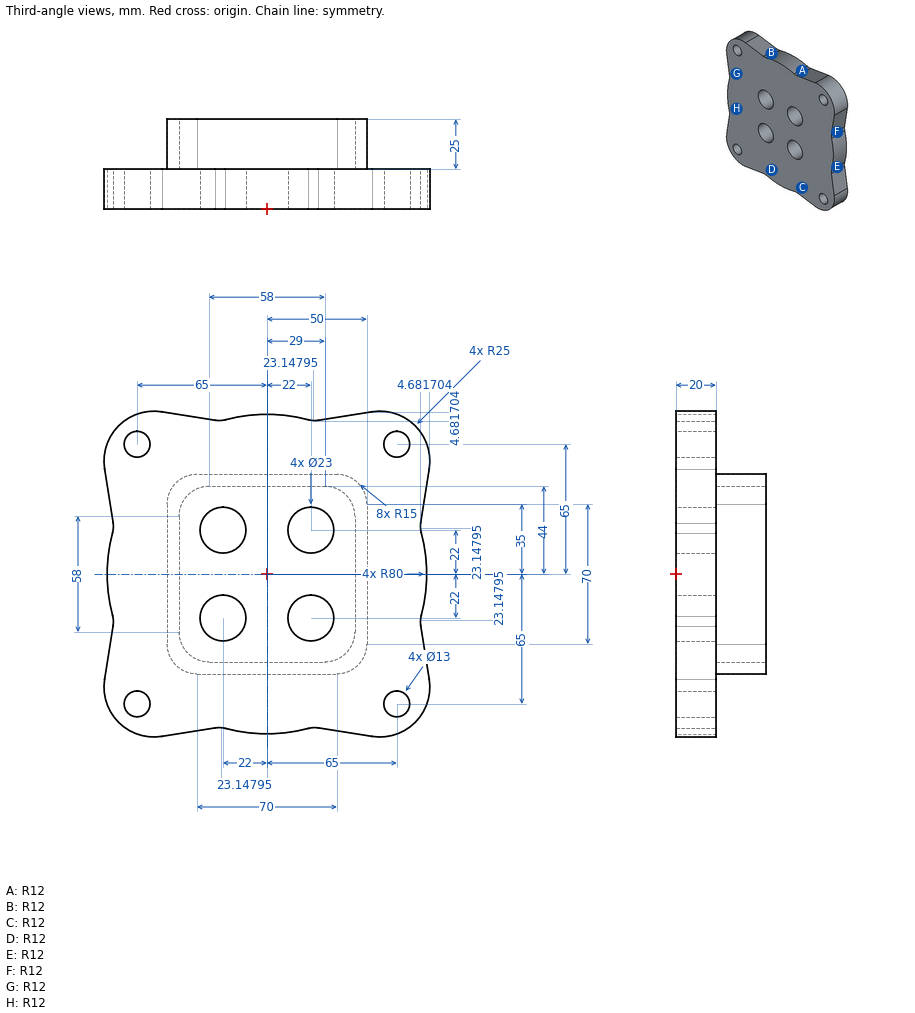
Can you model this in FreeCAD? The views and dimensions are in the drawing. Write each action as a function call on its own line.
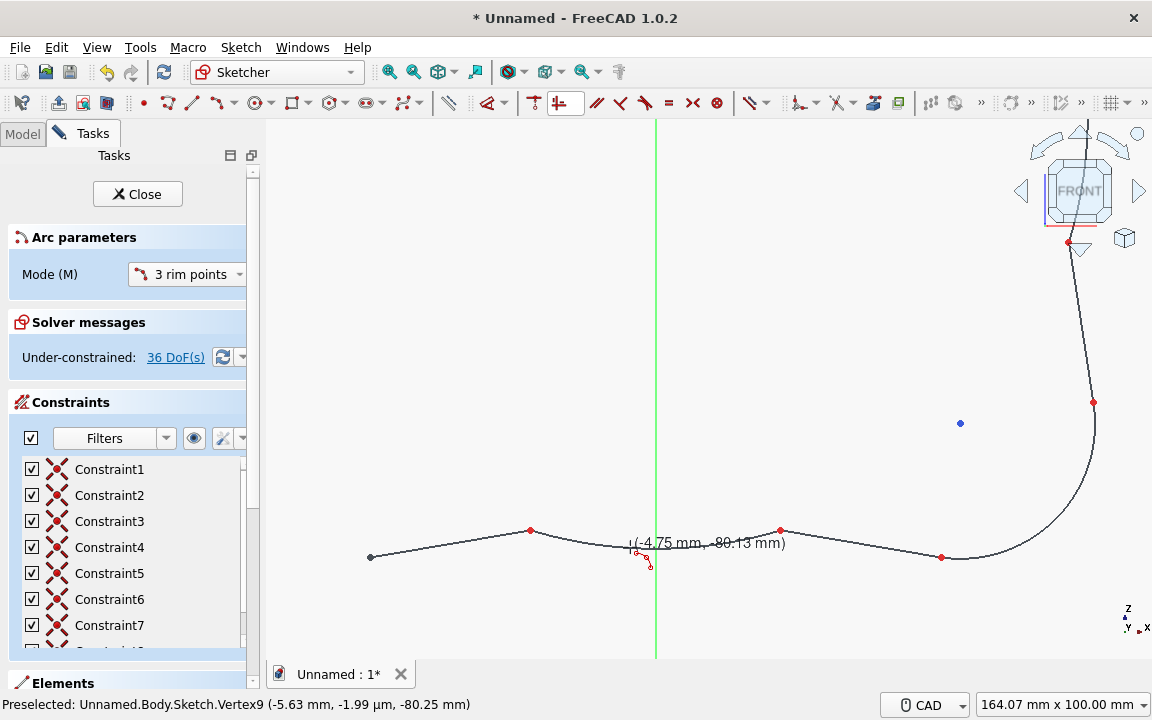
click(370, 558)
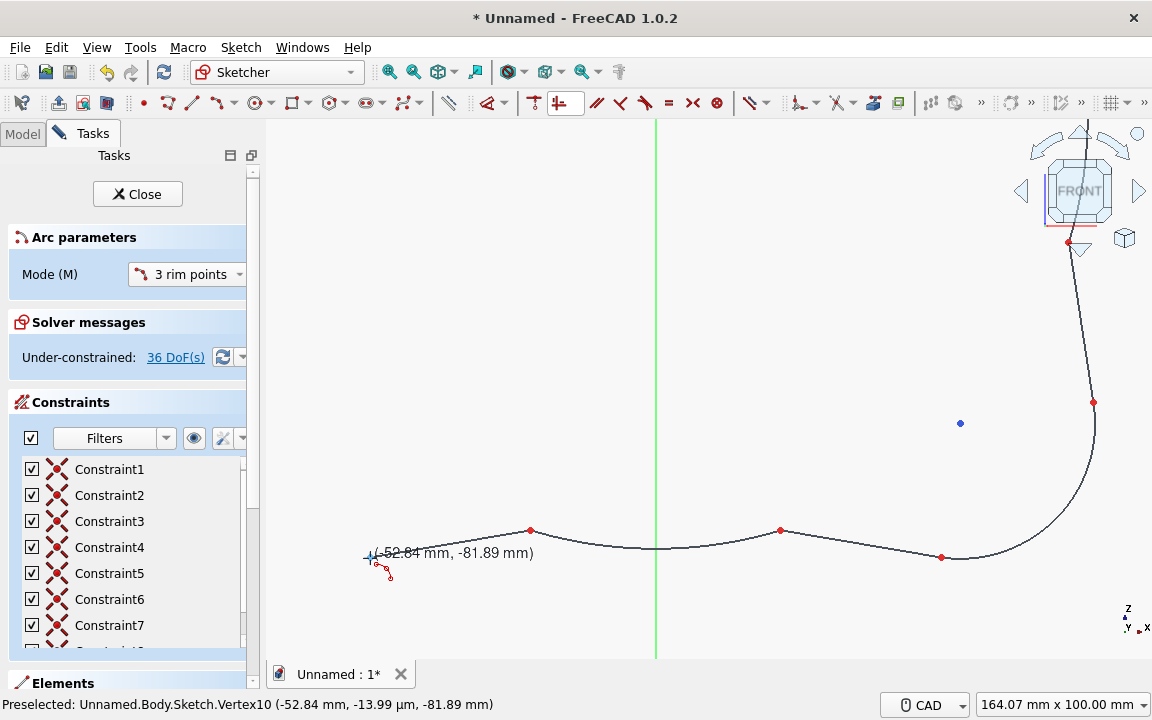
scroll(632, 548, down, 5)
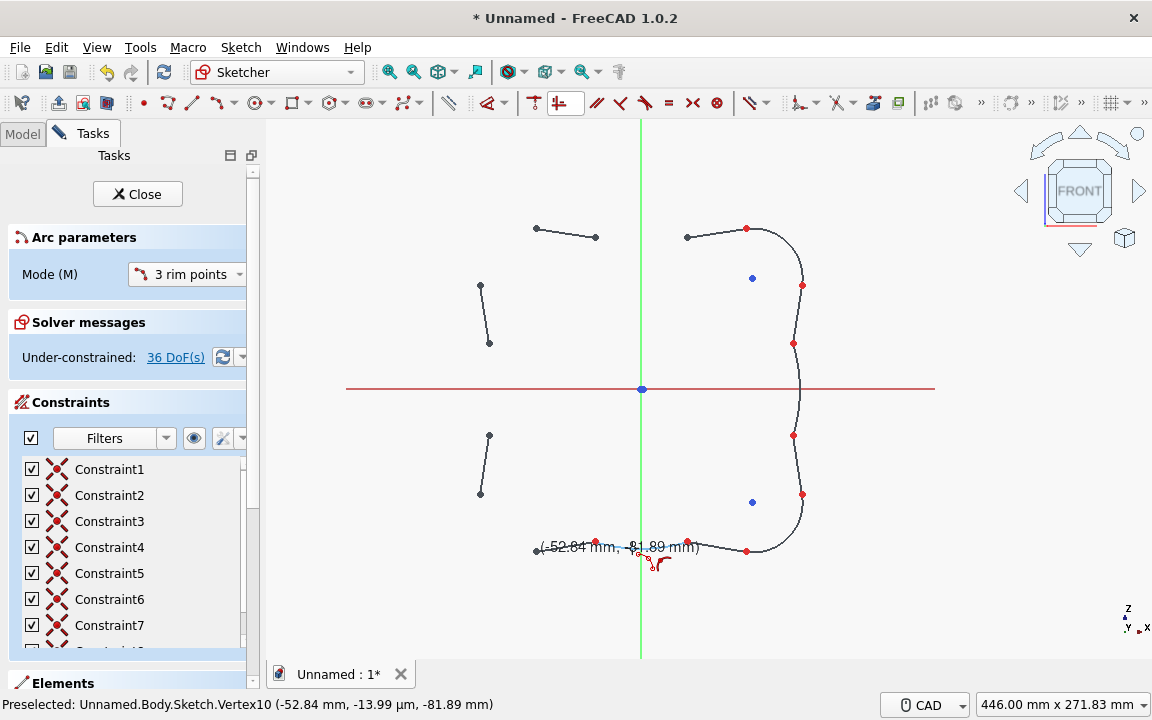
click(480, 495)
click(493, 537)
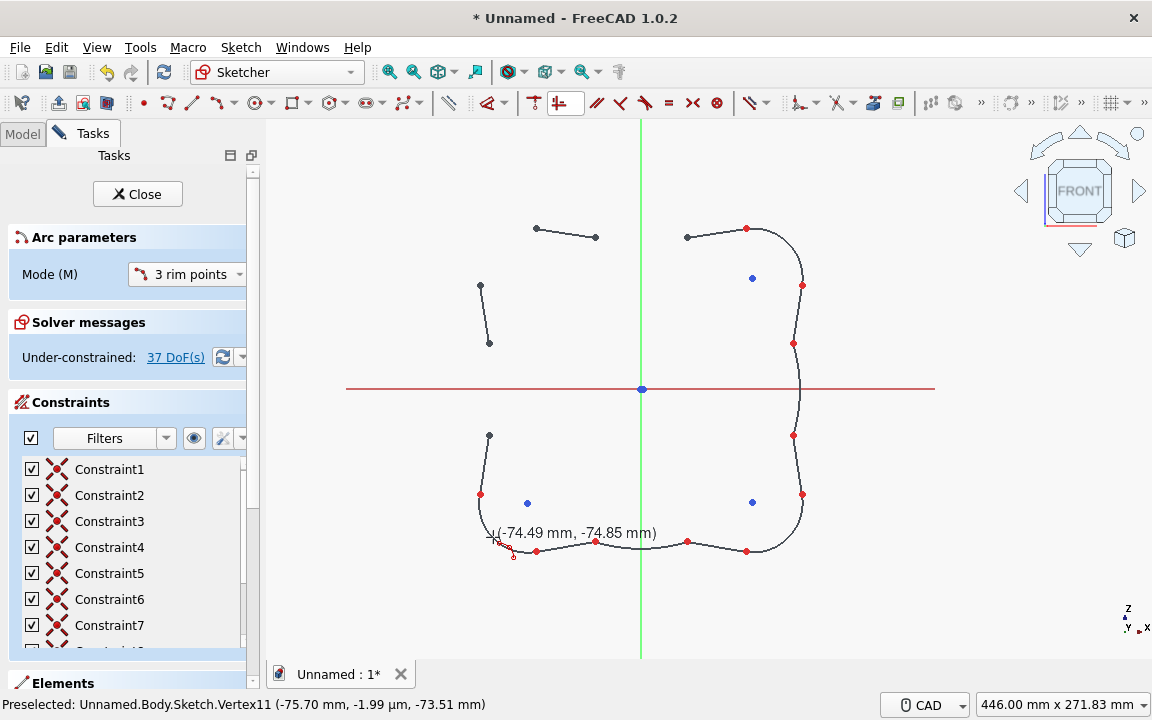
click(489, 436)
click(489, 344)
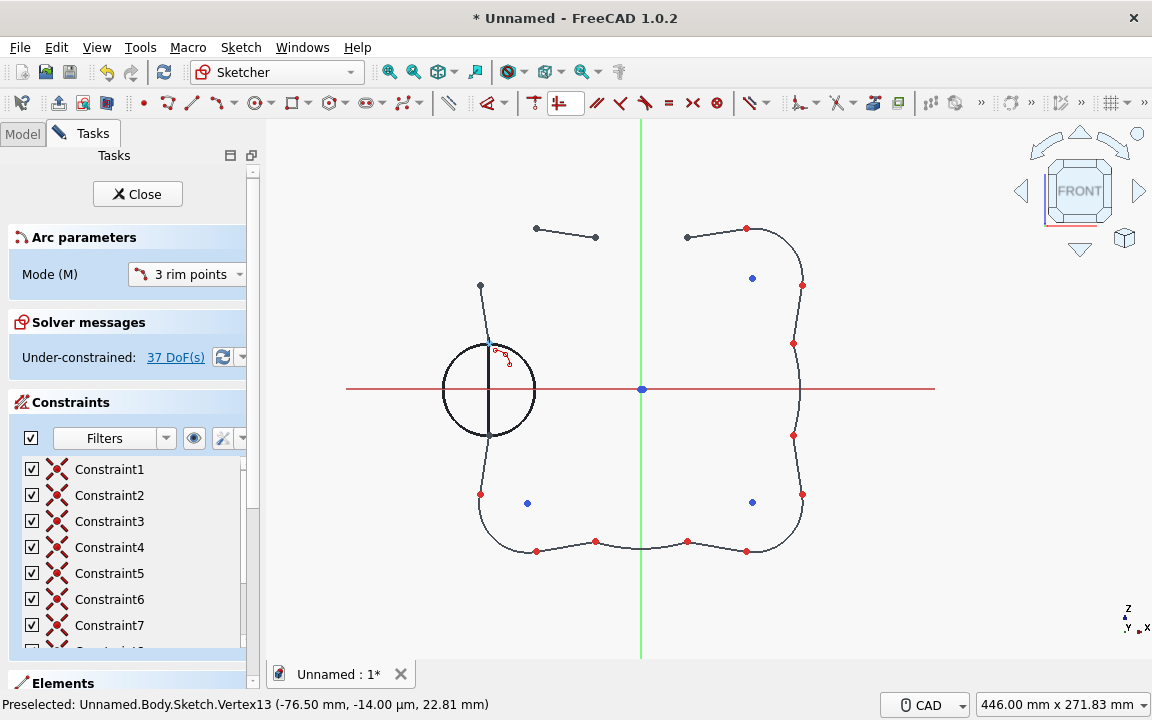
scroll(482, 380, up, 5)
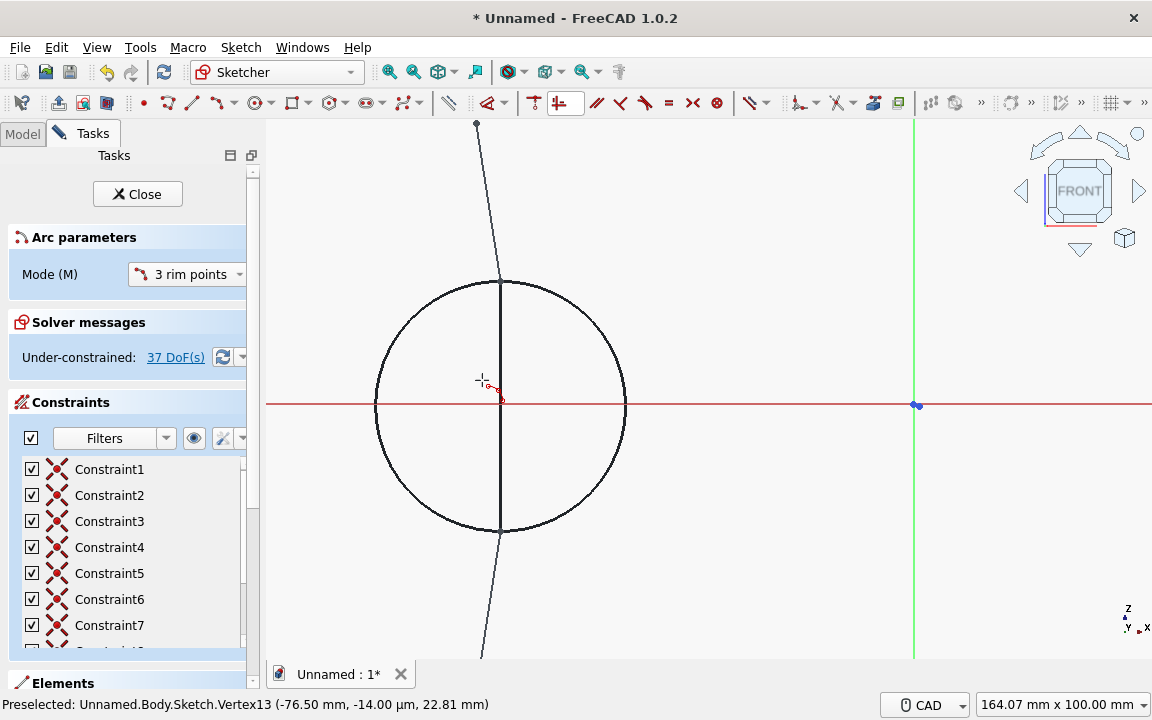
click(482, 379)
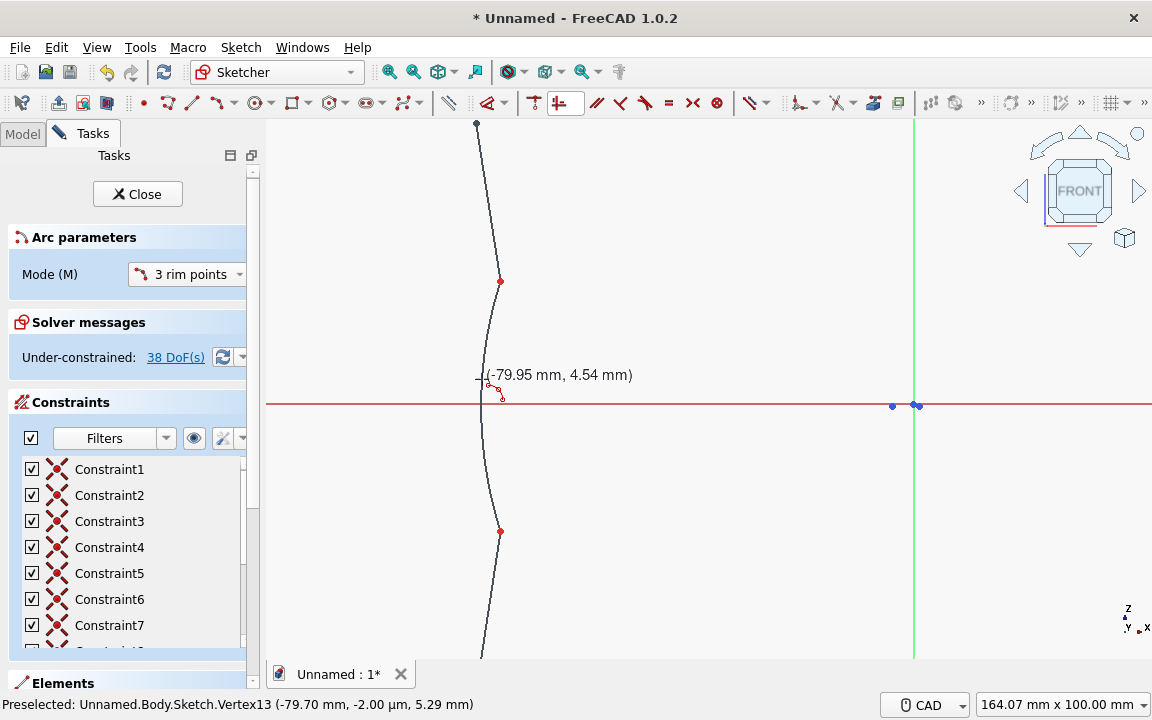
scroll(482, 380, down, 5)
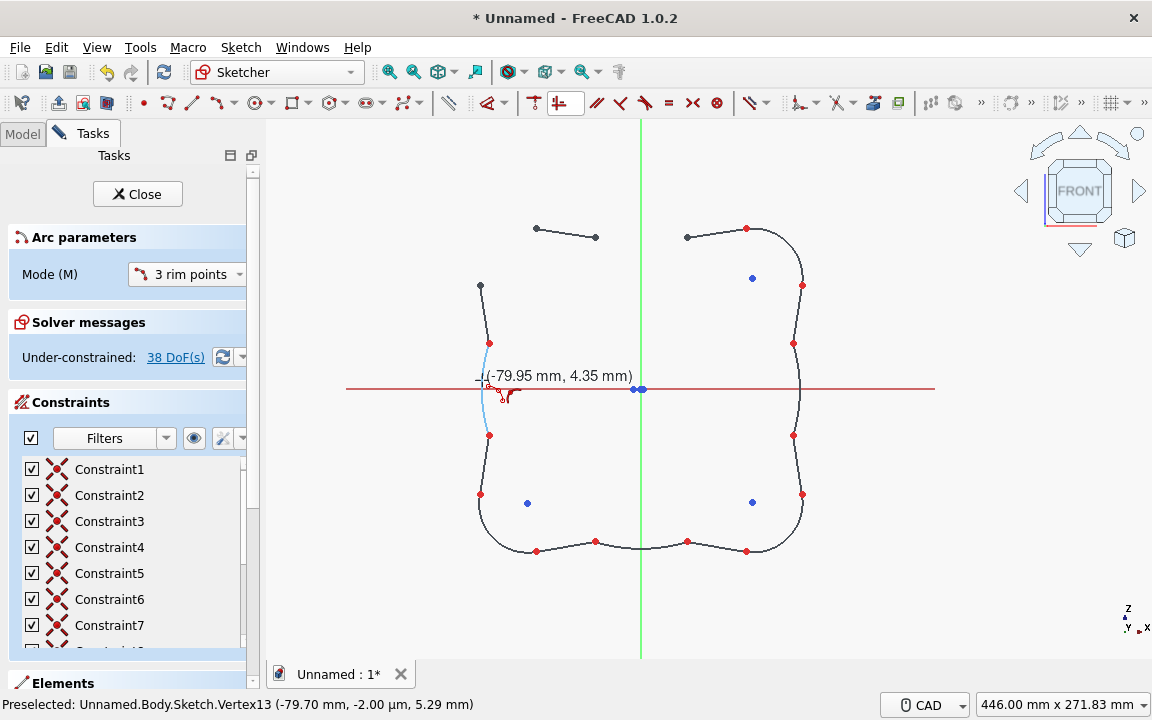
click(480, 286)
click(536, 229)
click(493, 242)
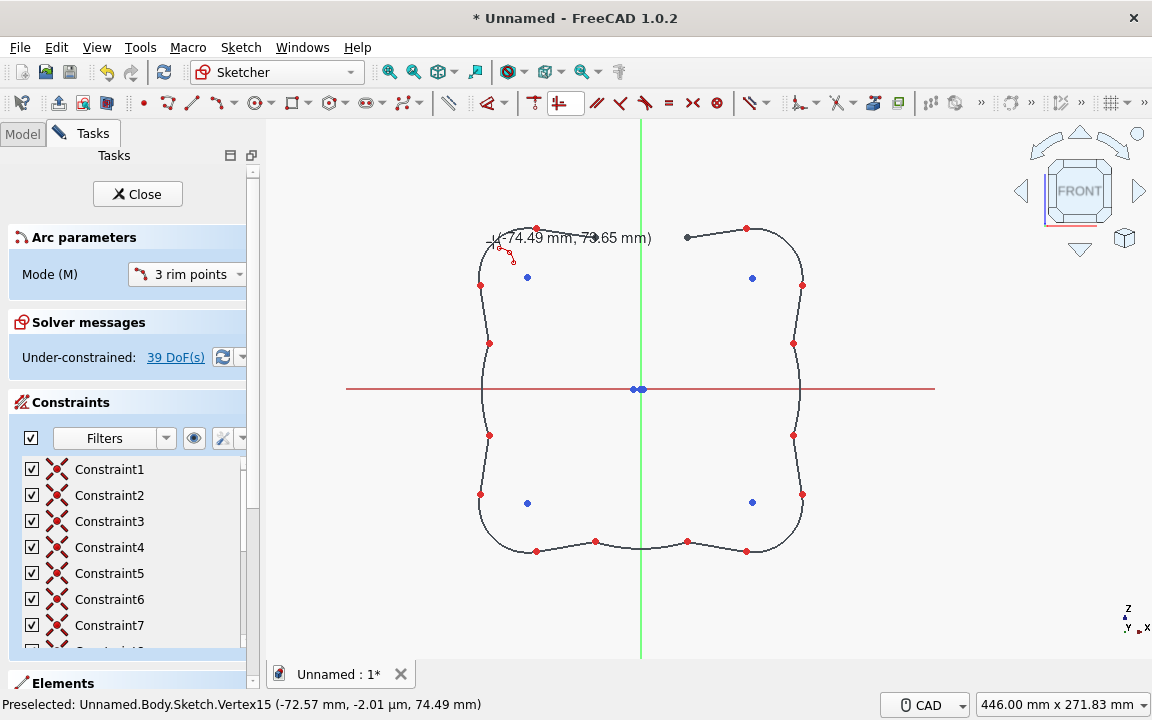
click(595, 238)
click(687, 238)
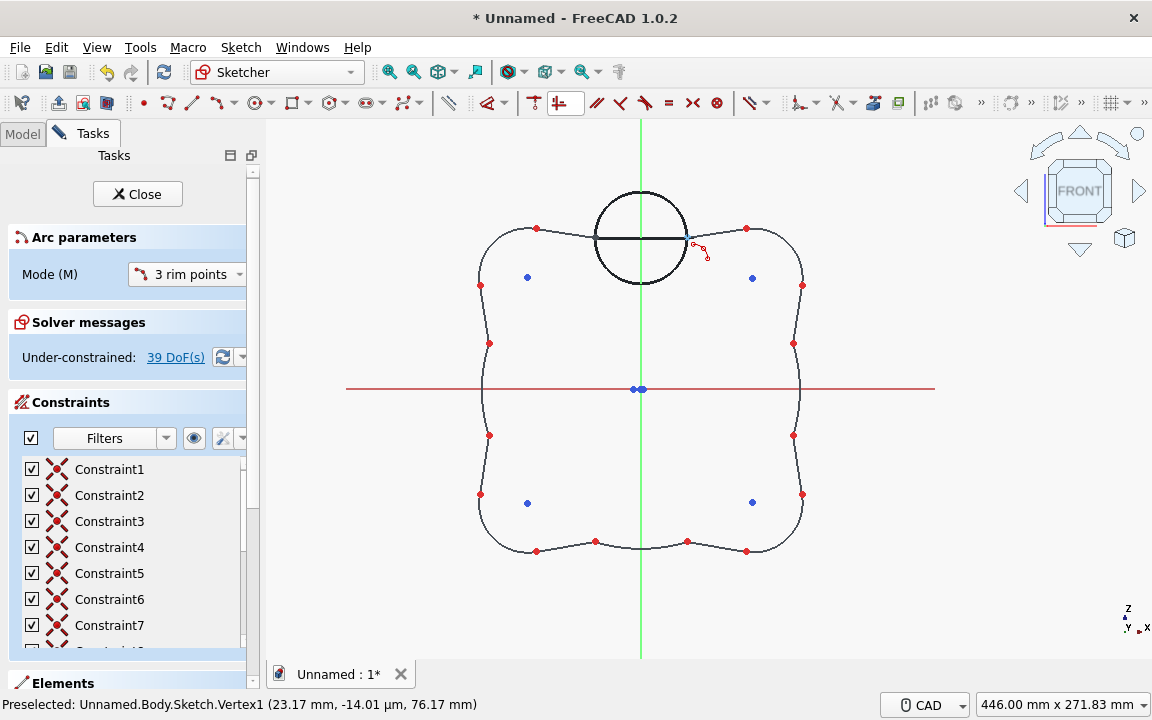
scroll(650, 231, up, 5)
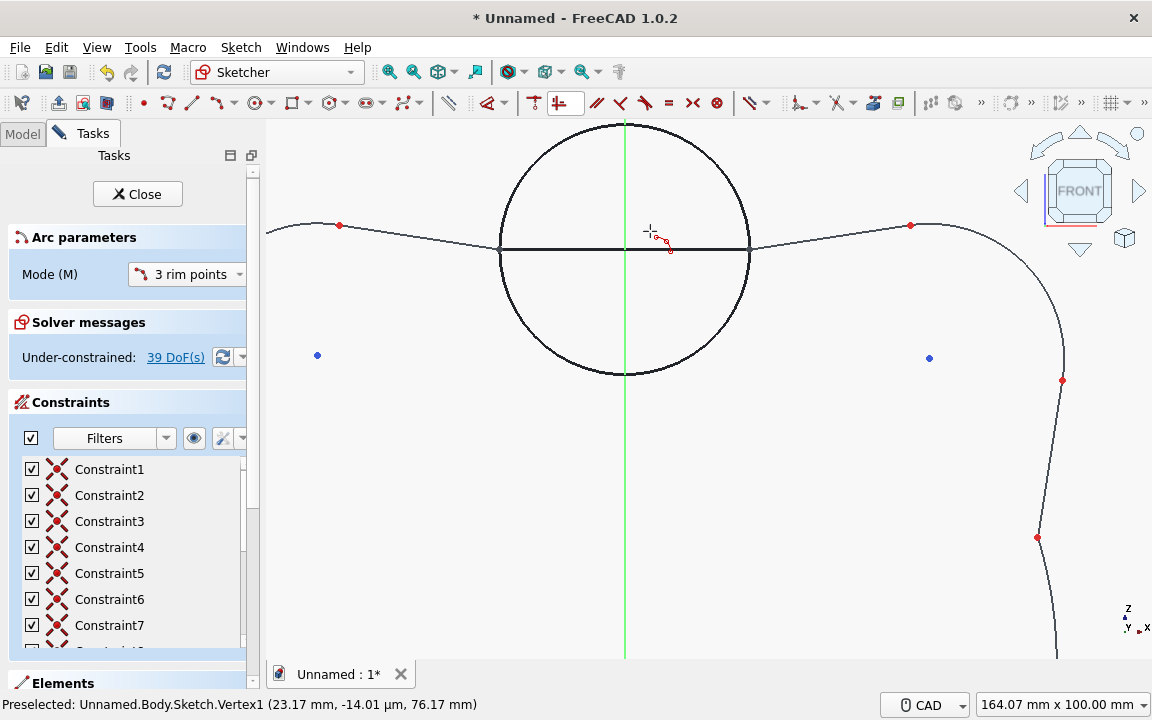
click(650, 230)
key(Escape)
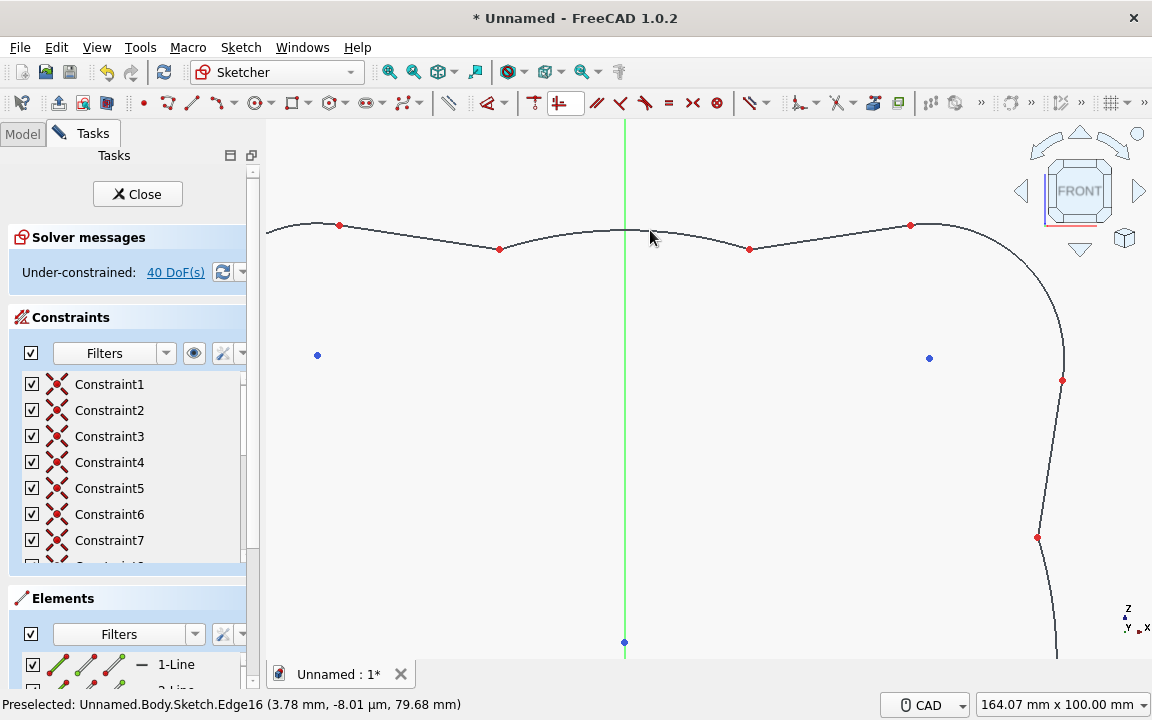
click(798, 242)